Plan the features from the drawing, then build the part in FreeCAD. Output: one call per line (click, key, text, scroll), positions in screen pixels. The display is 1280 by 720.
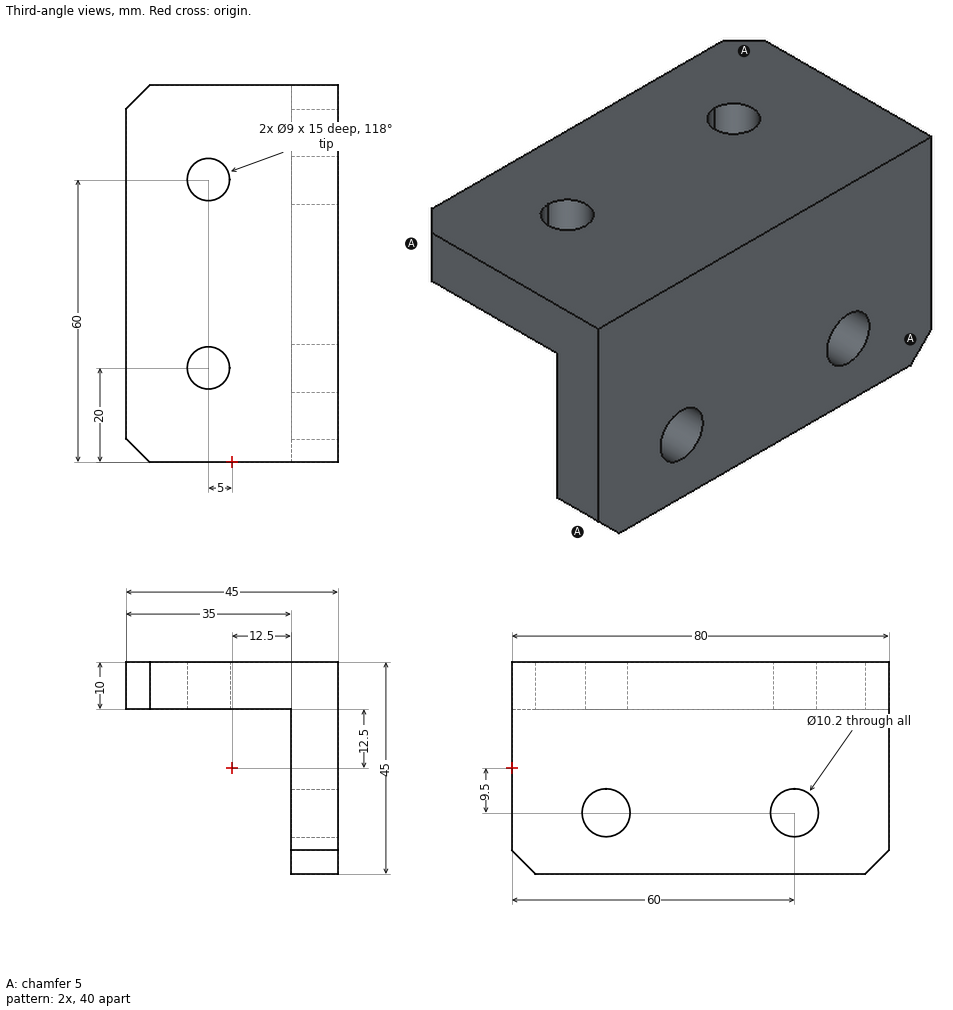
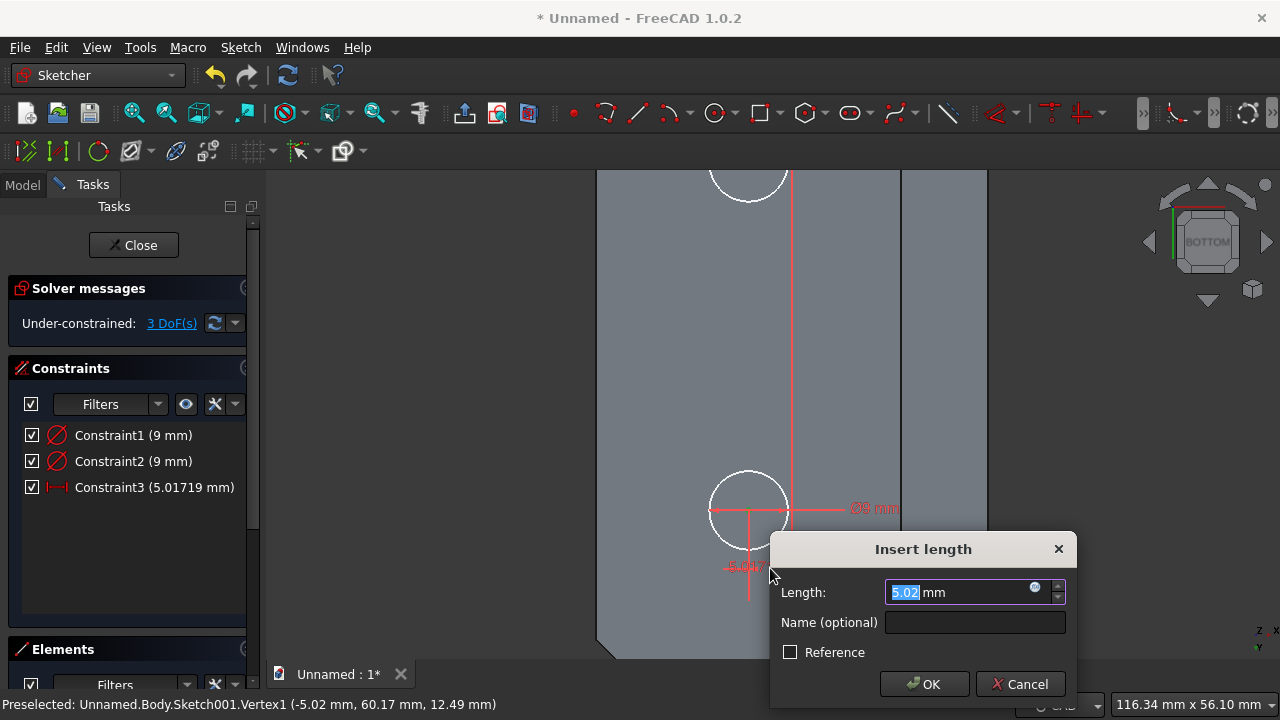
text(5)
key(Return)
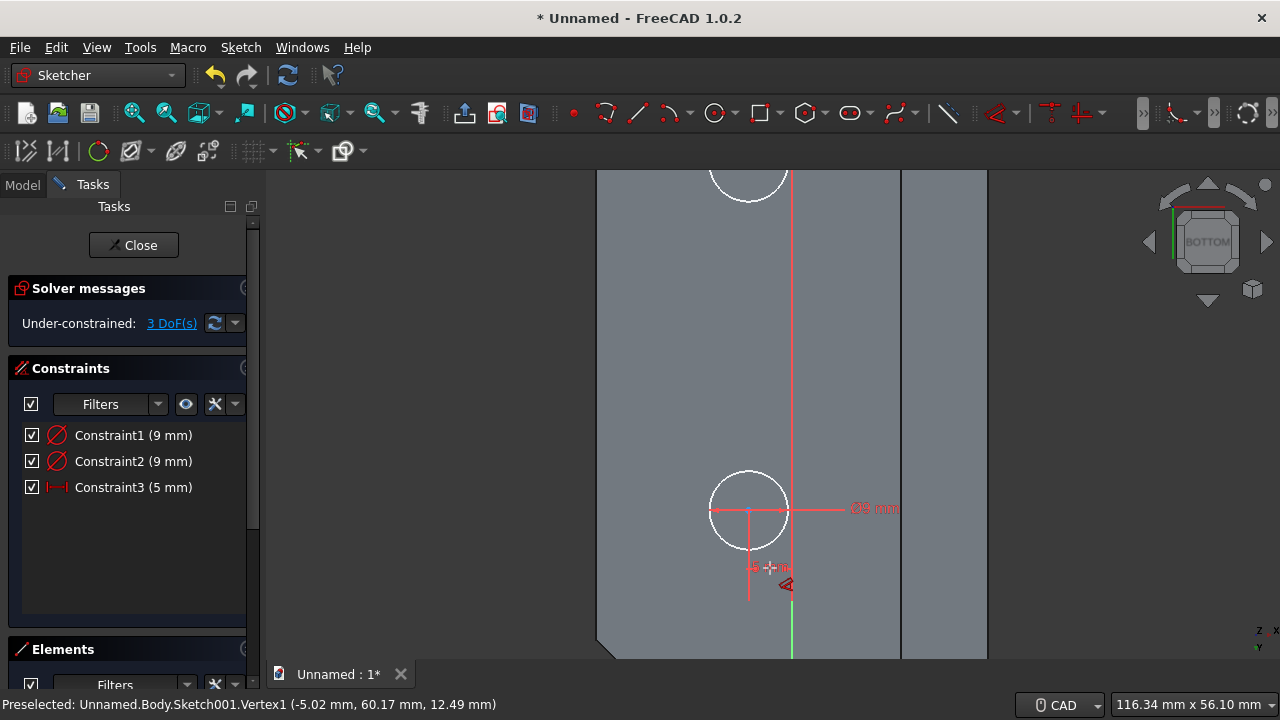
scroll(648, 594, down, 3)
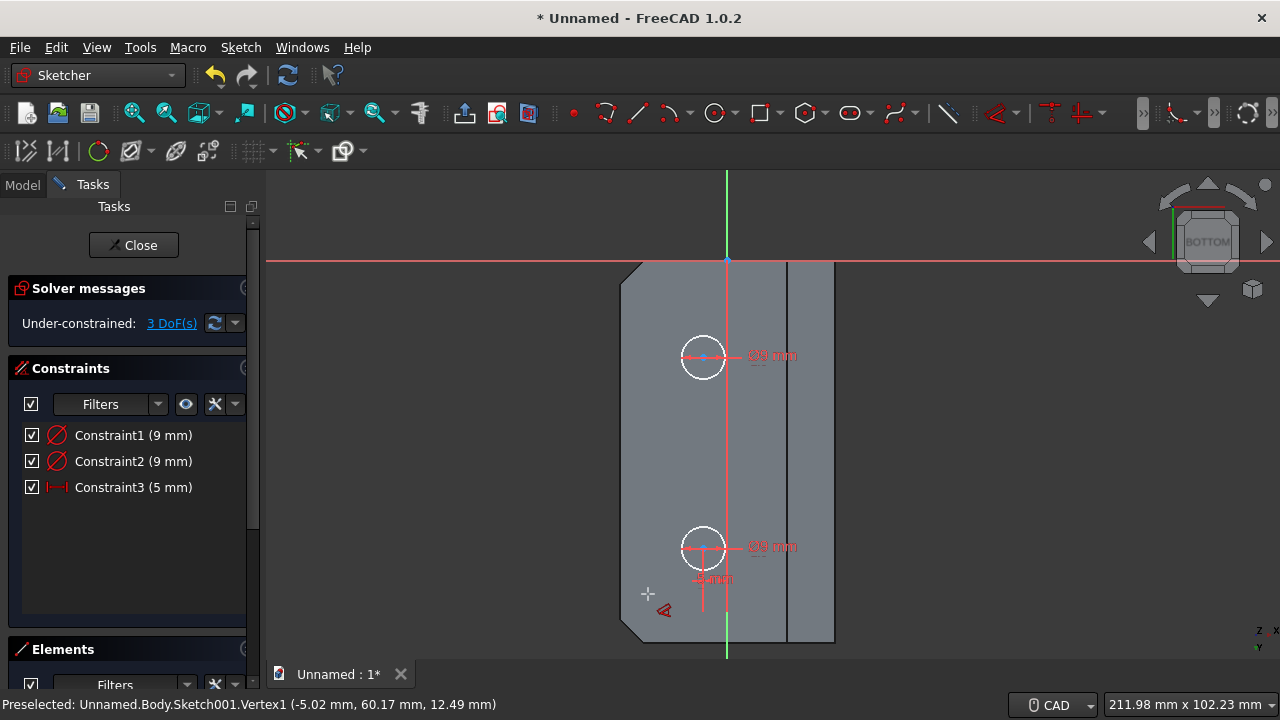
scroll(703, 358, up, 3)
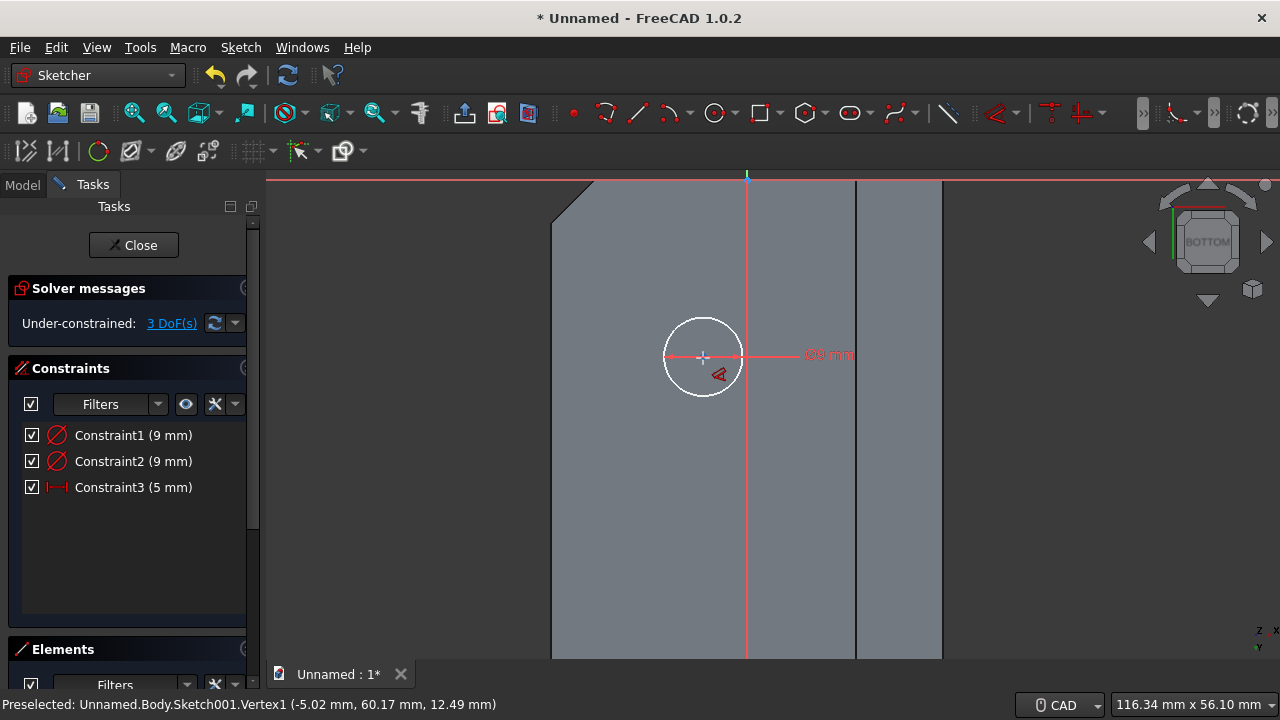
click(703, 357)
click(725, 415)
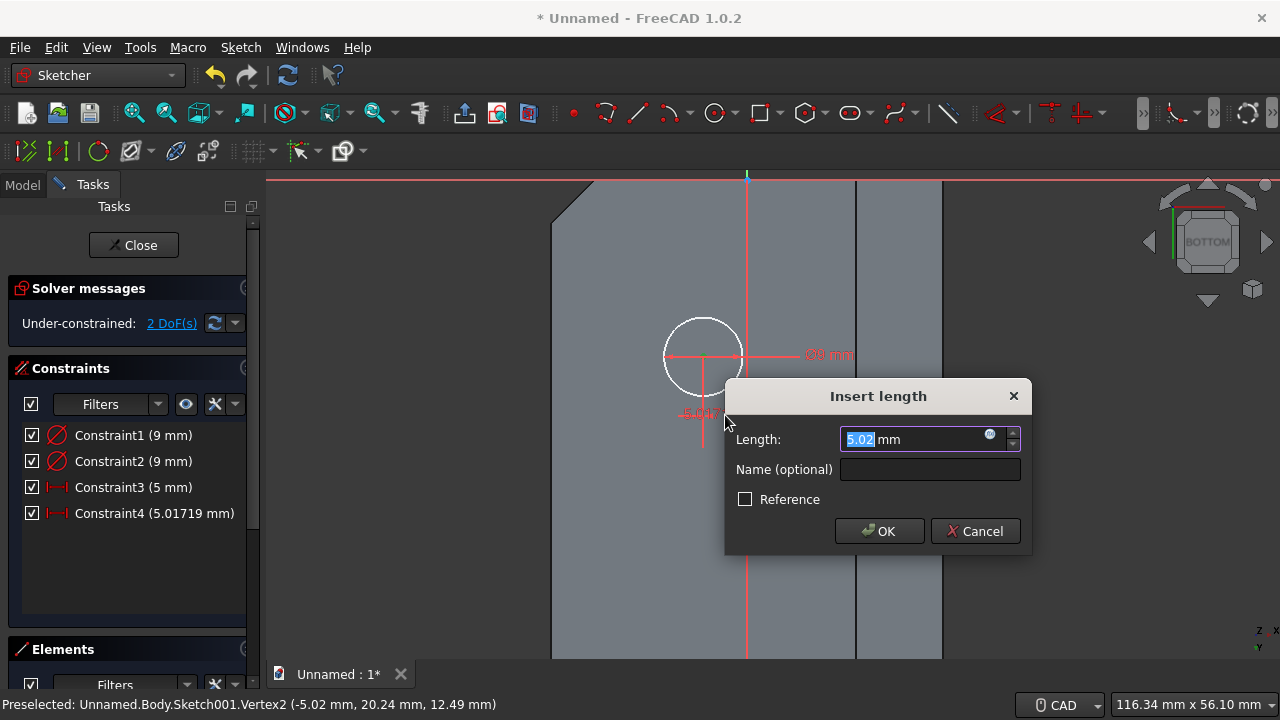
text(5)
key(Return)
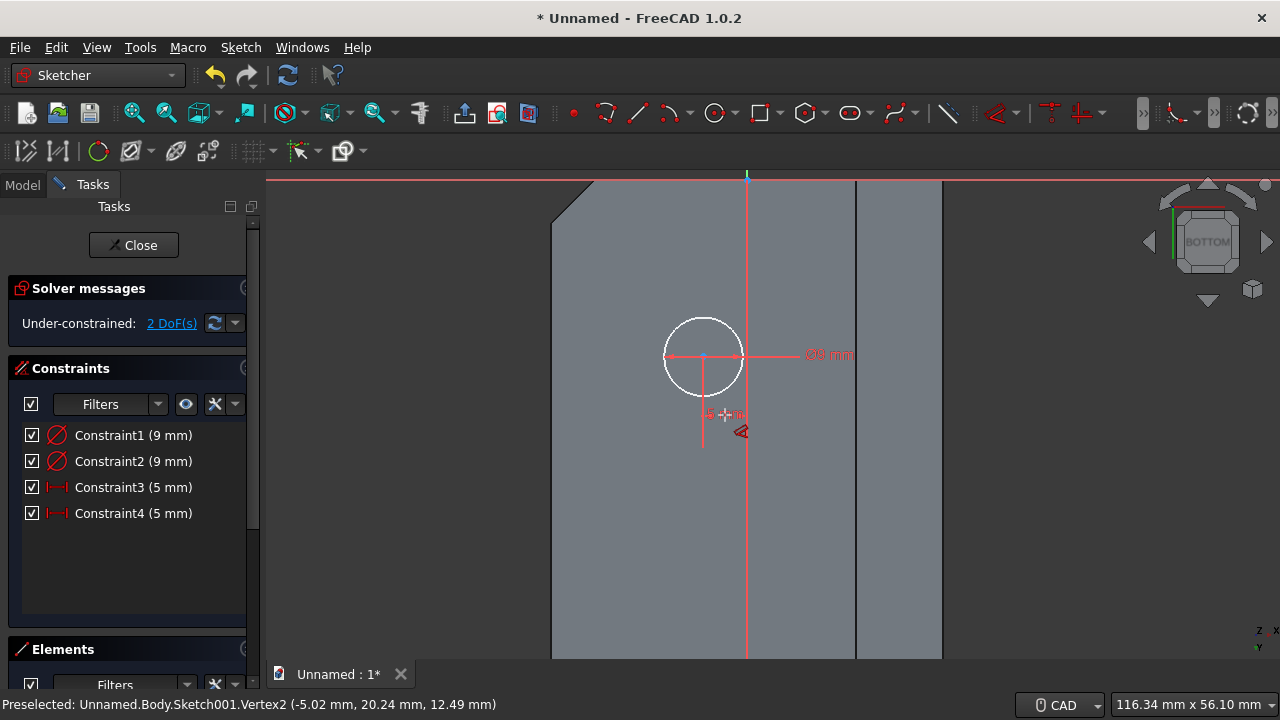
scroll(703, 357, down, 3)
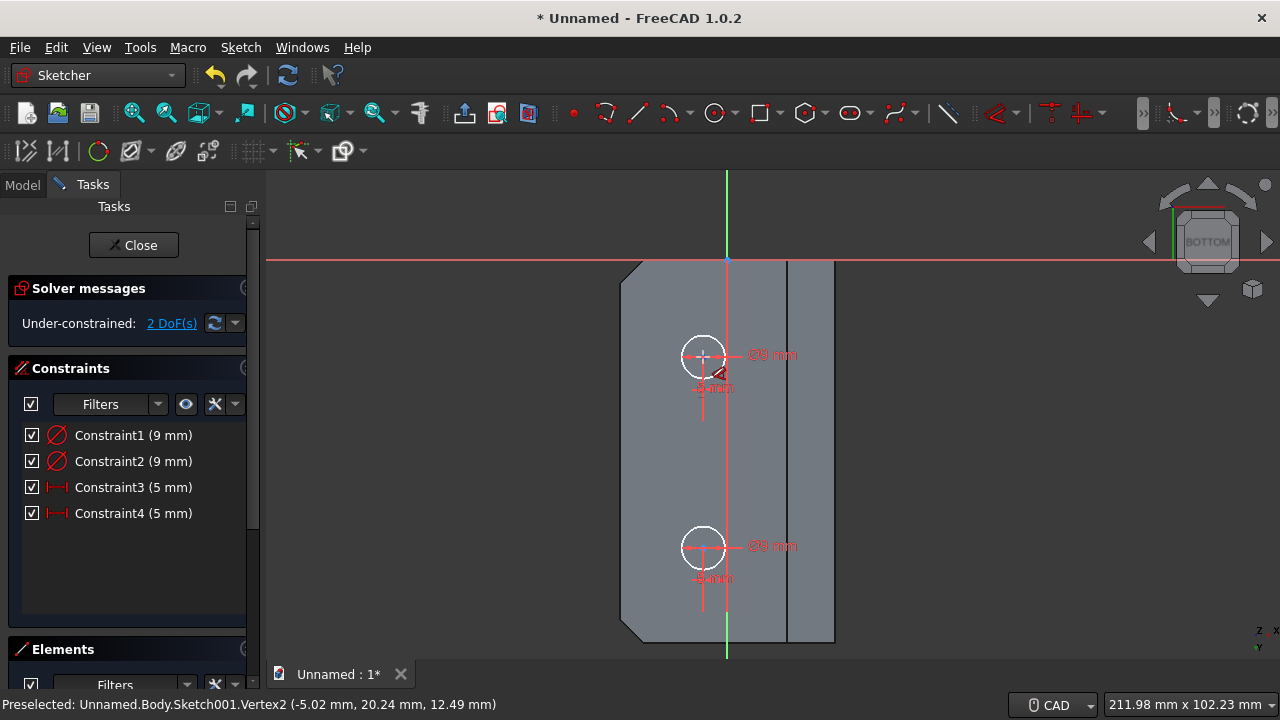
click(703, 548)
click(761, 338)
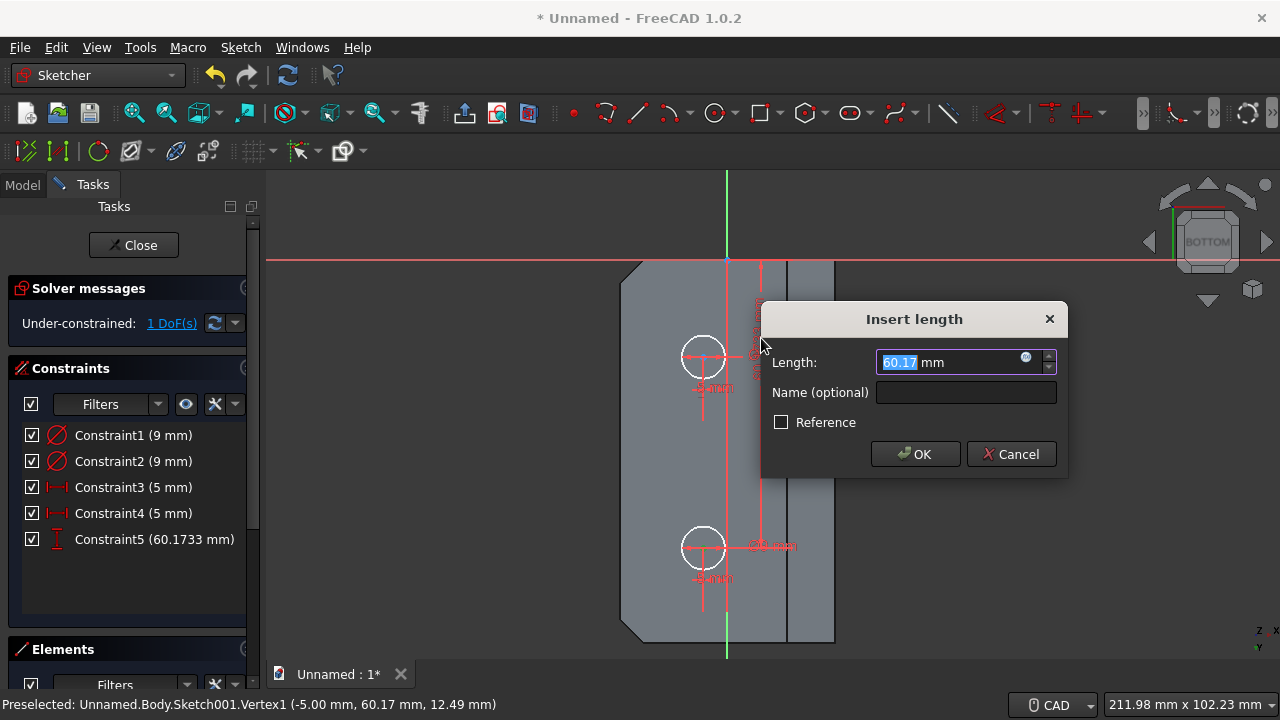
text(60)
key(Return)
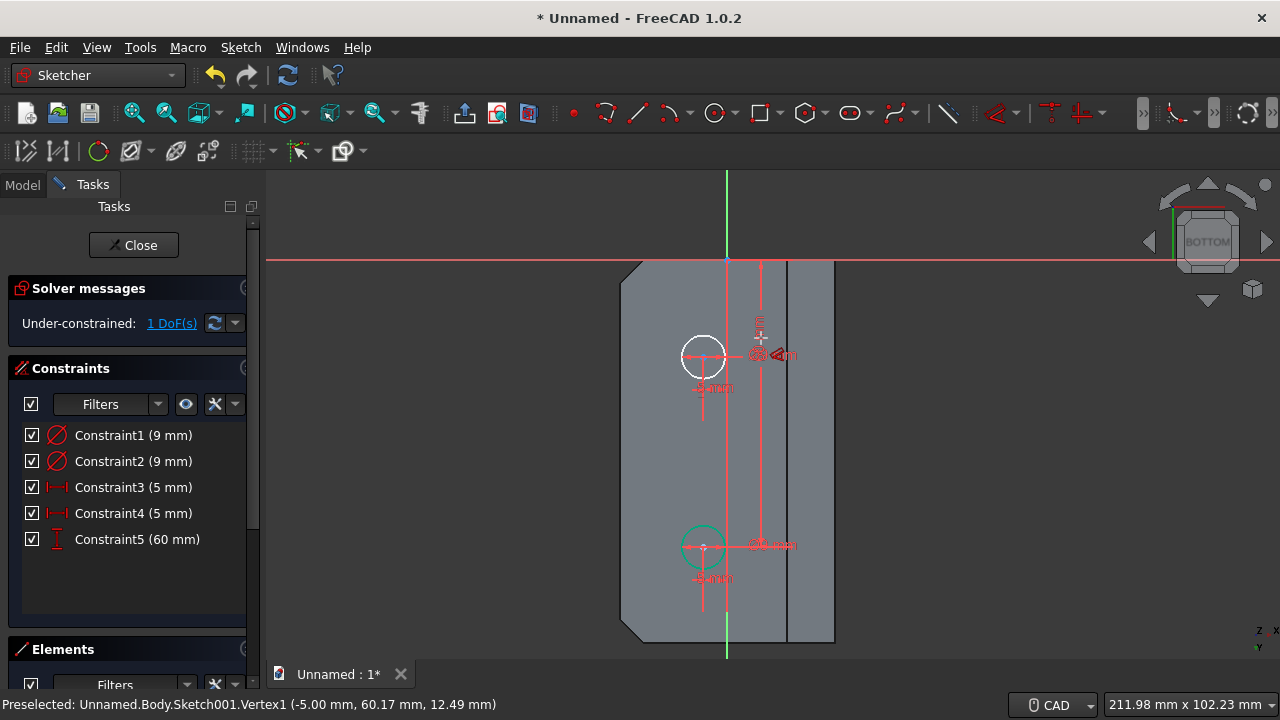
click(703, 357)
click(761, 309)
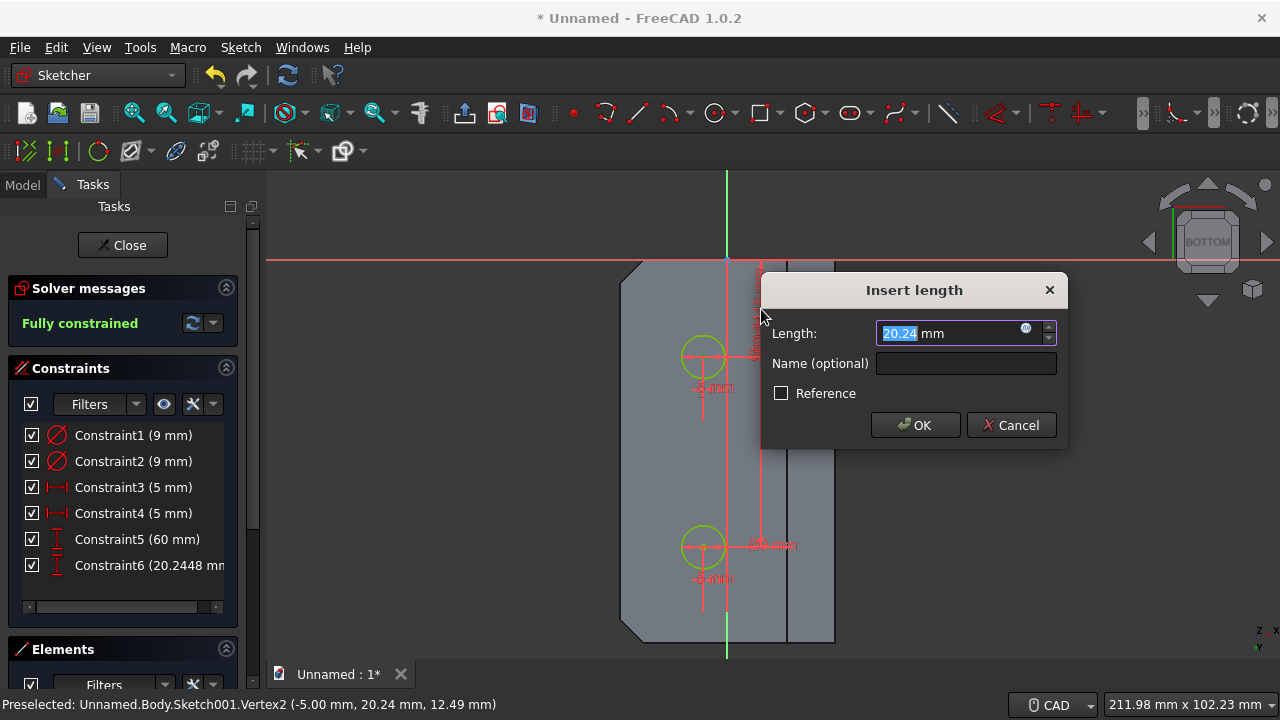
text(20)
key(Return)
key(Escape)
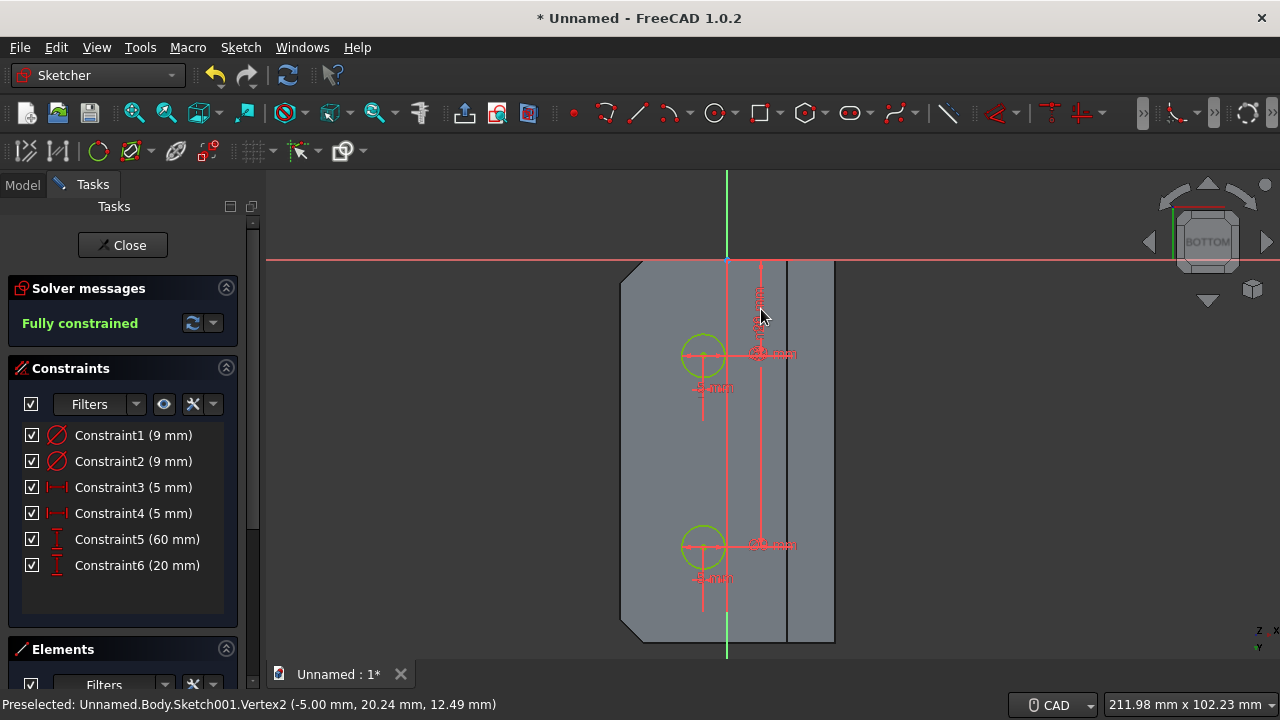
click(123, 245)